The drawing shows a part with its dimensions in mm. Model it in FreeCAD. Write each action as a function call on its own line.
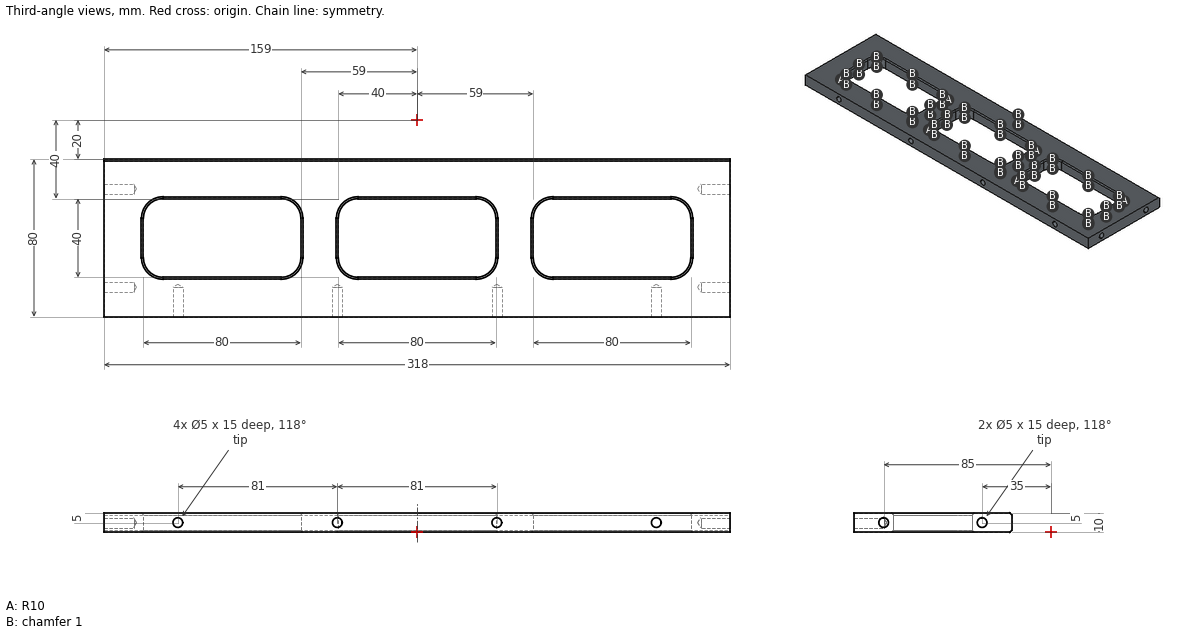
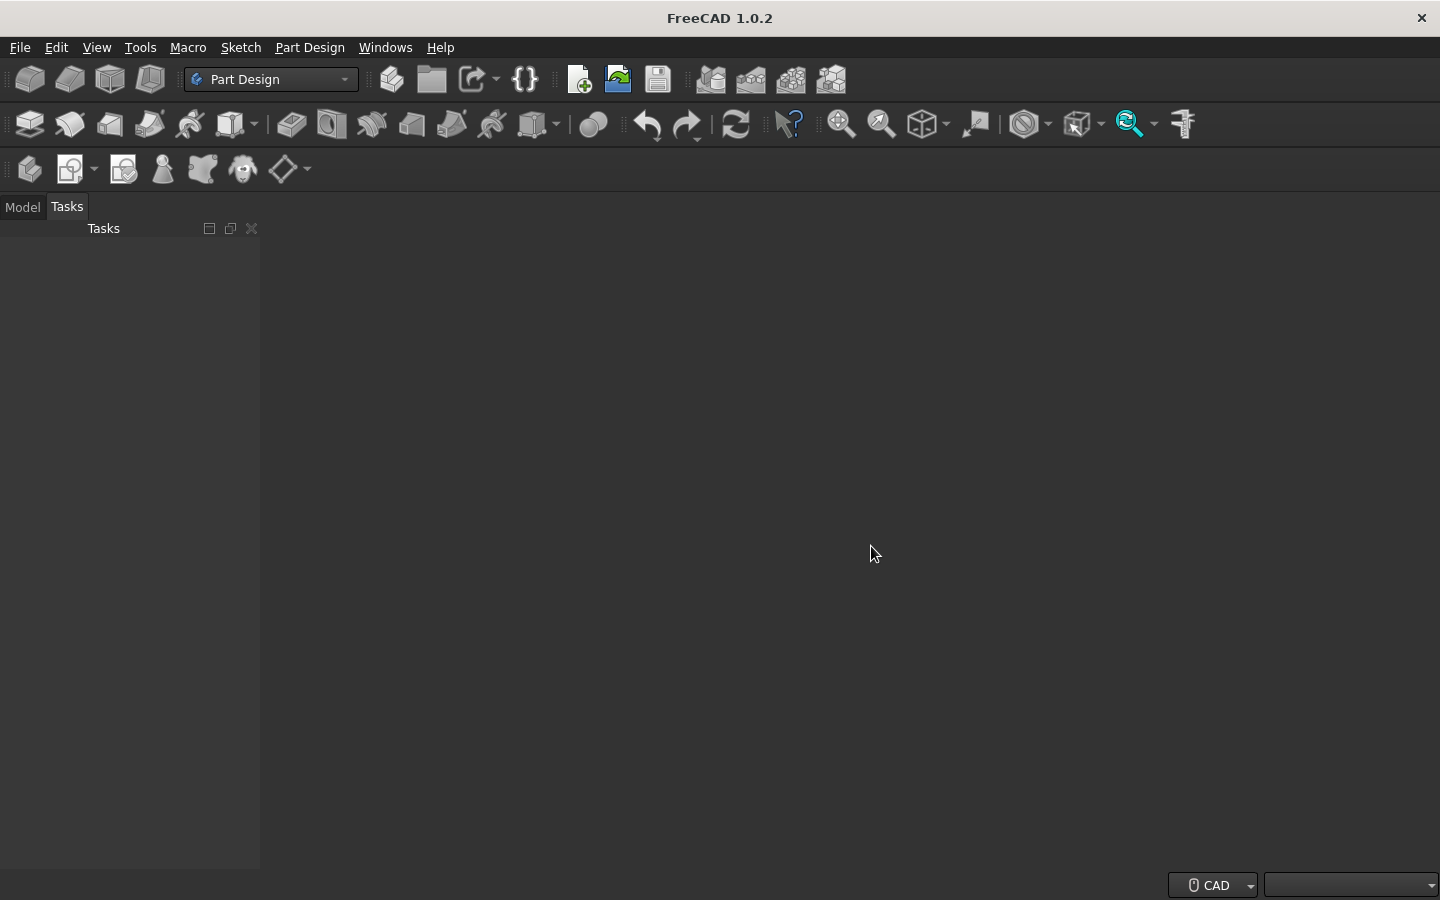
click(578, 80)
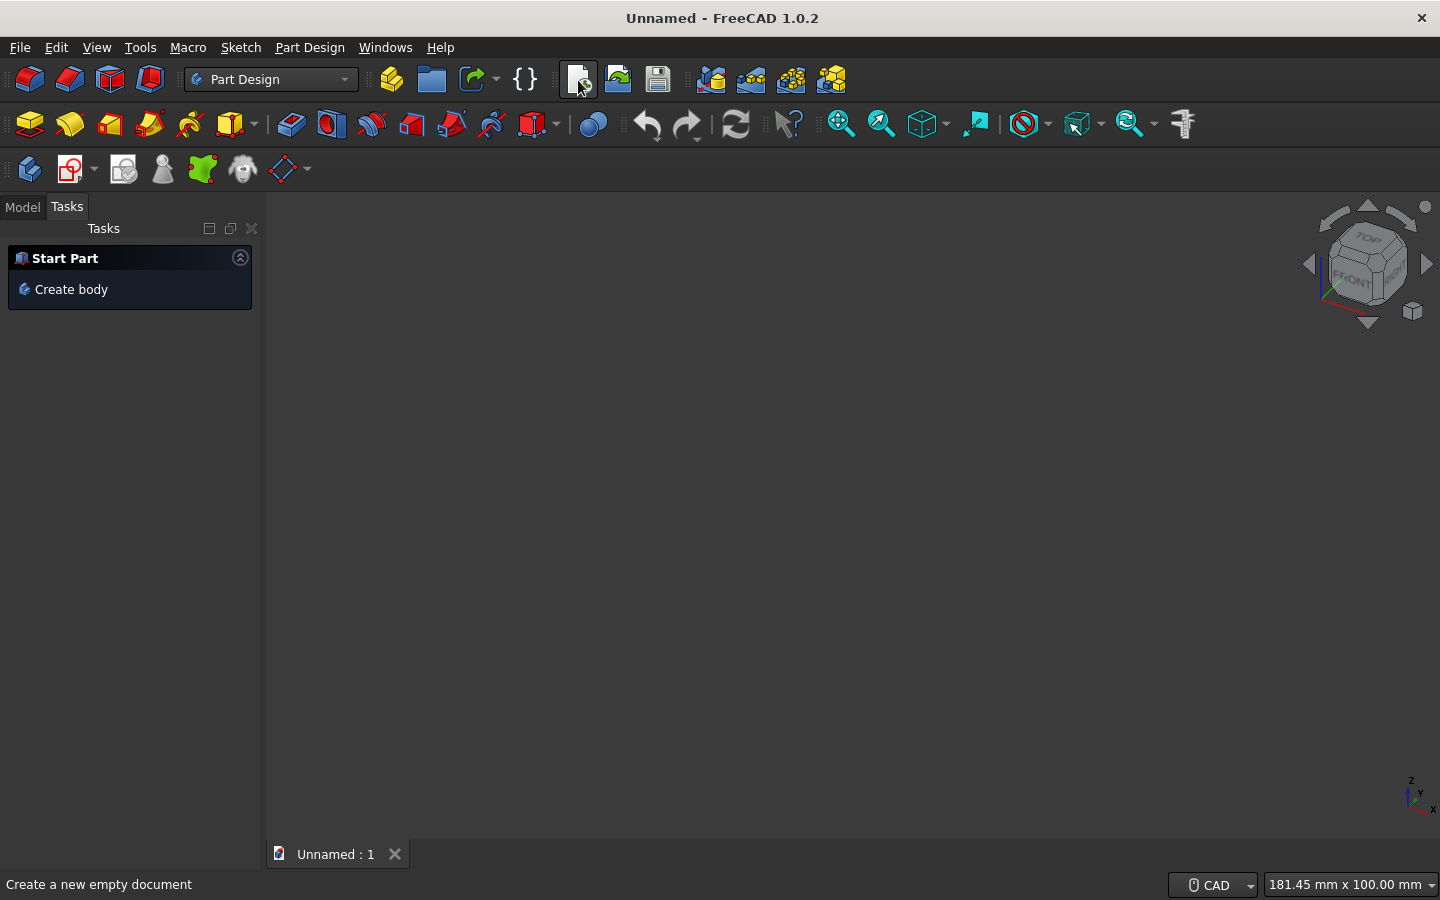
click(30, 170)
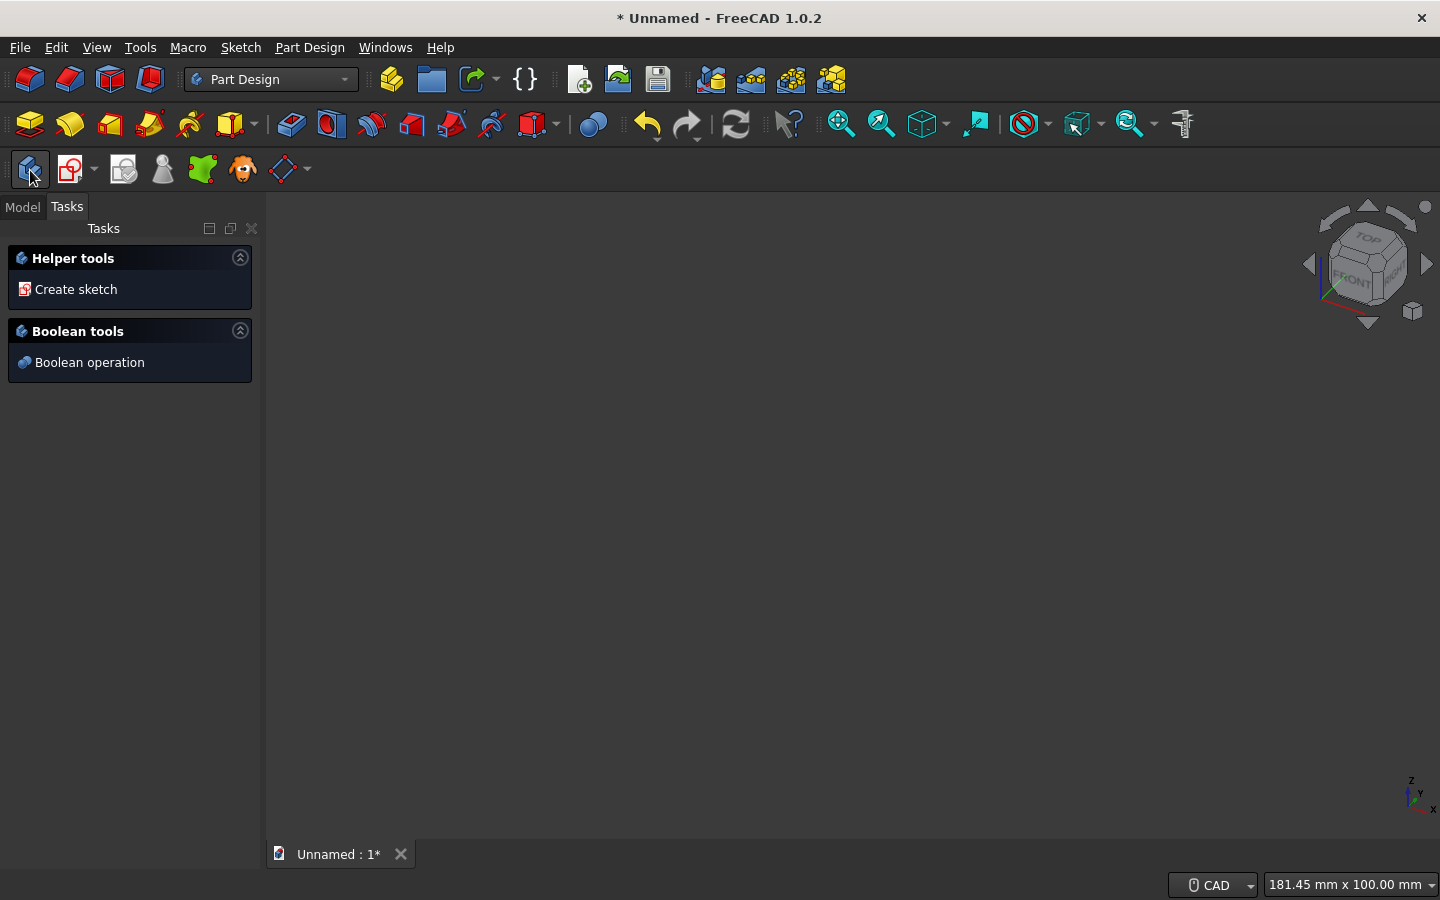
click(23, 206)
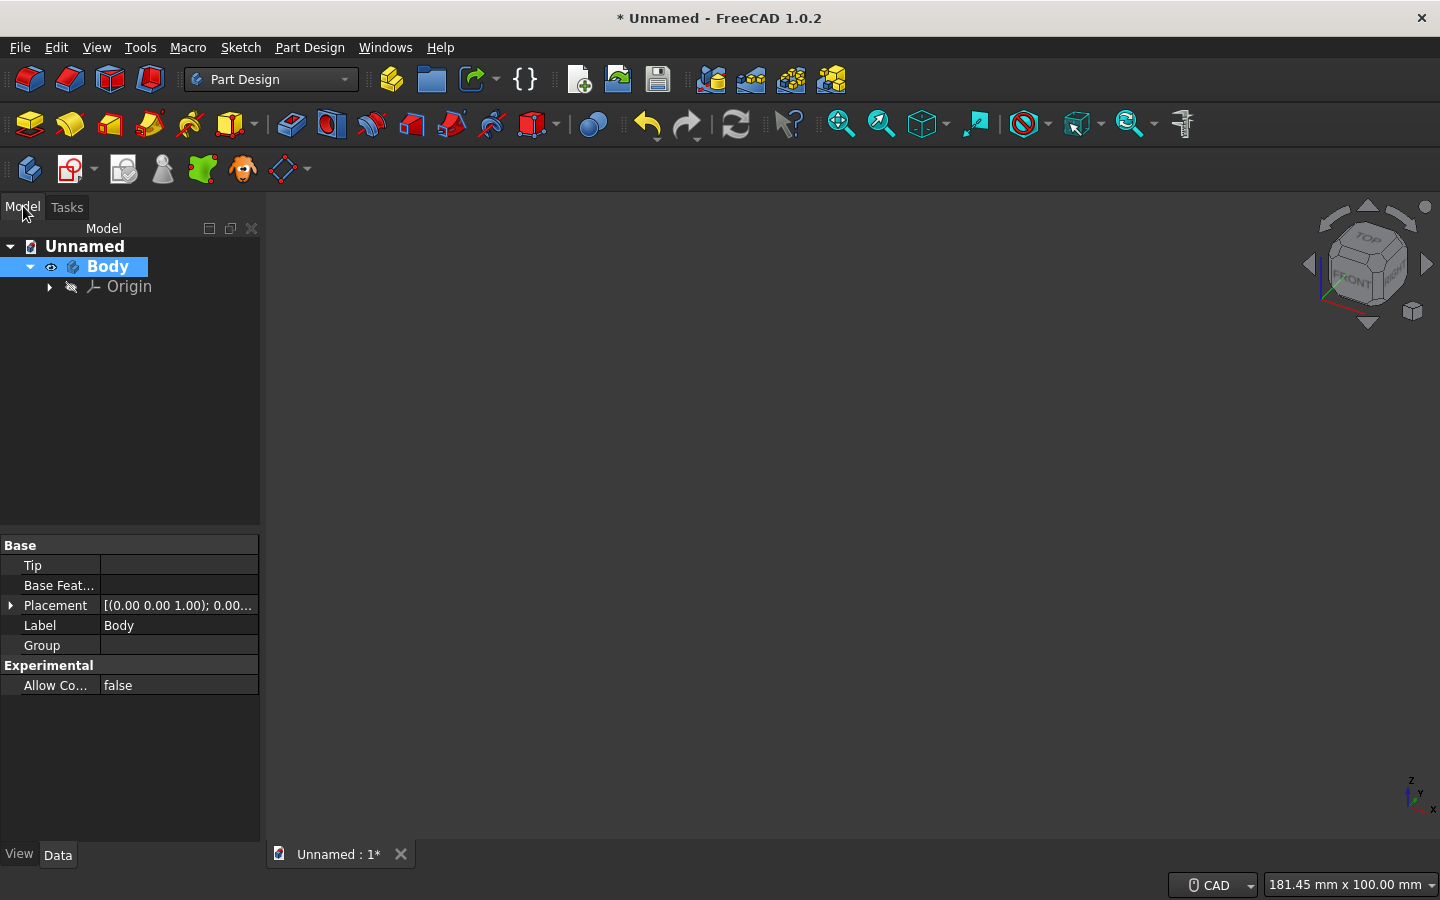
click(50, 287)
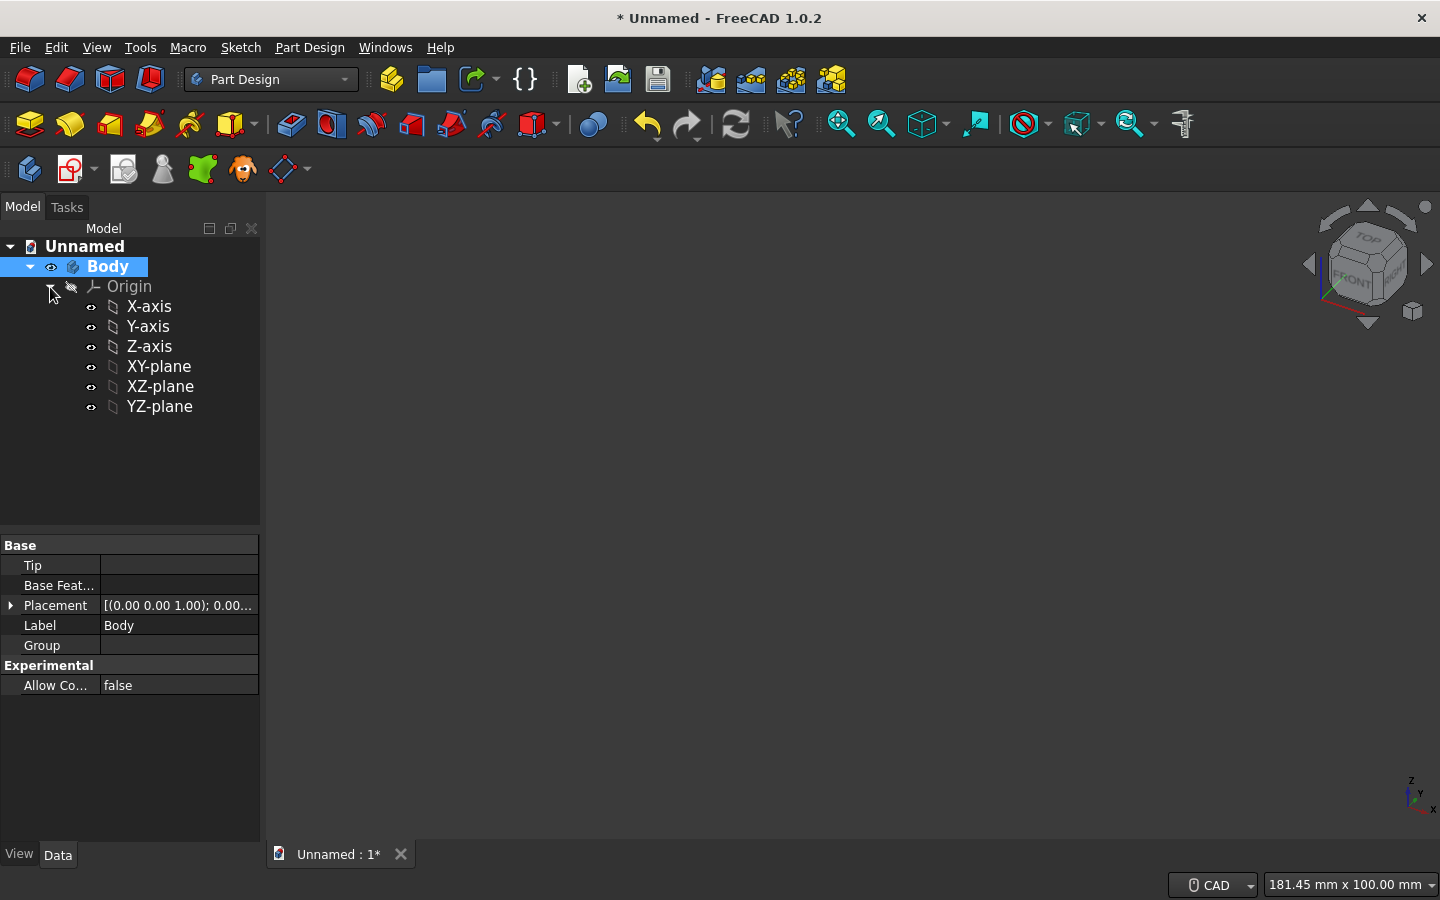
click(136, 367)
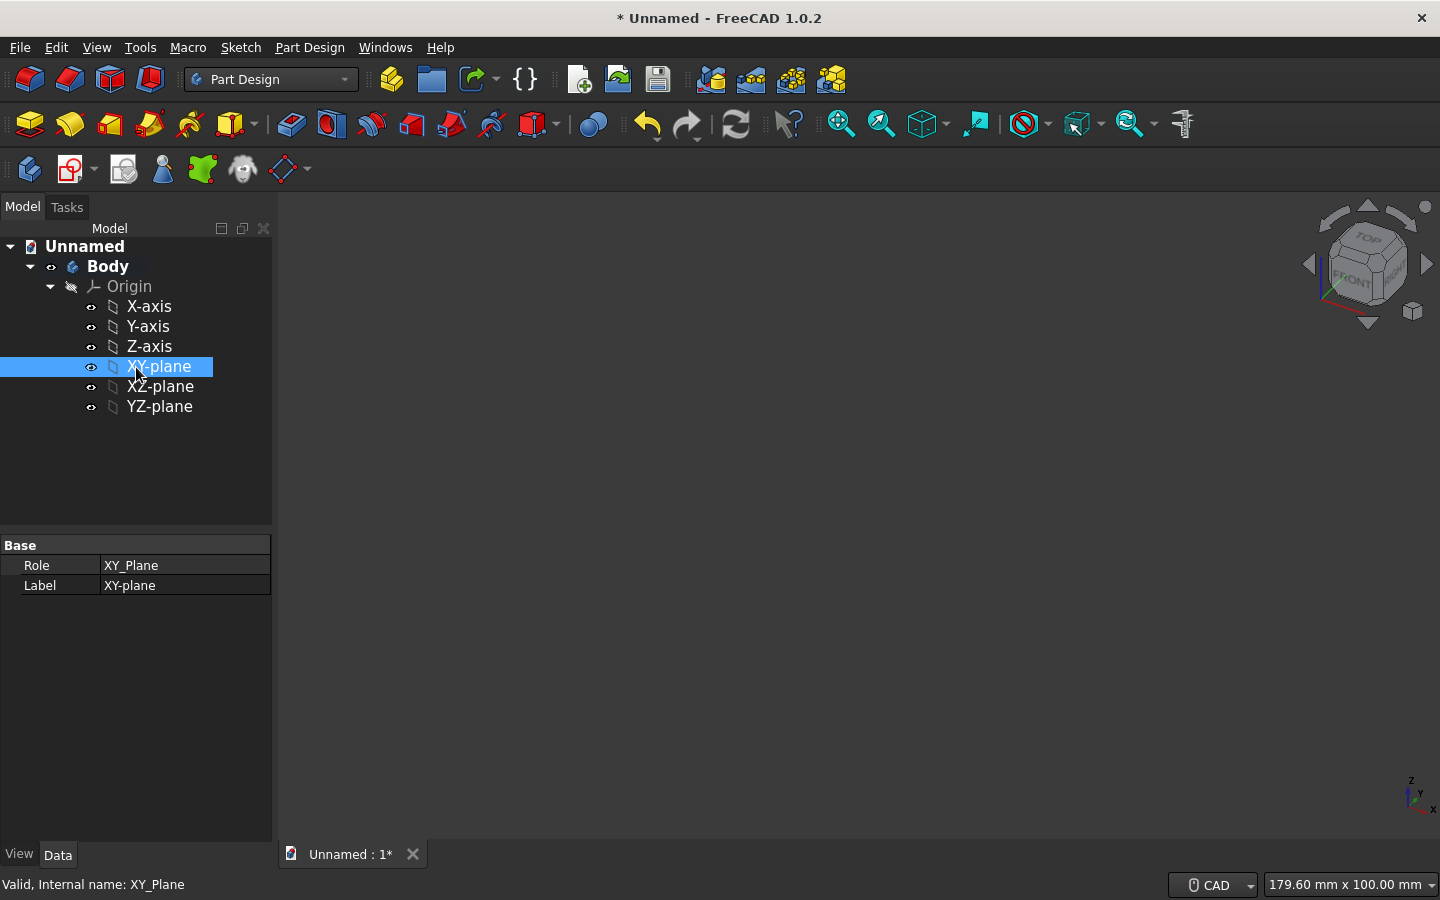
click(284, 170)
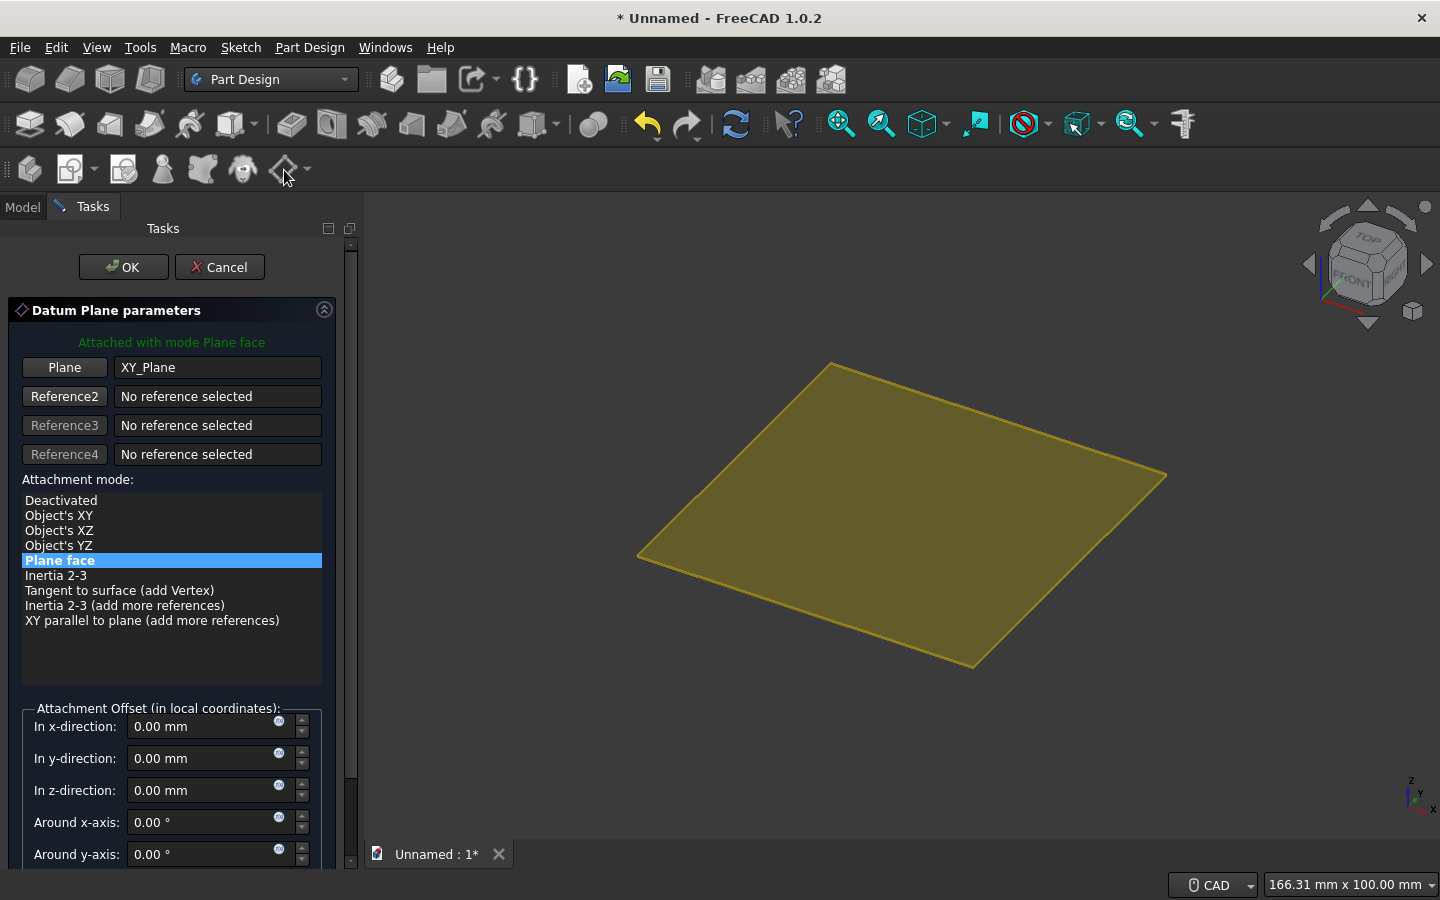
triple_click(210, 790)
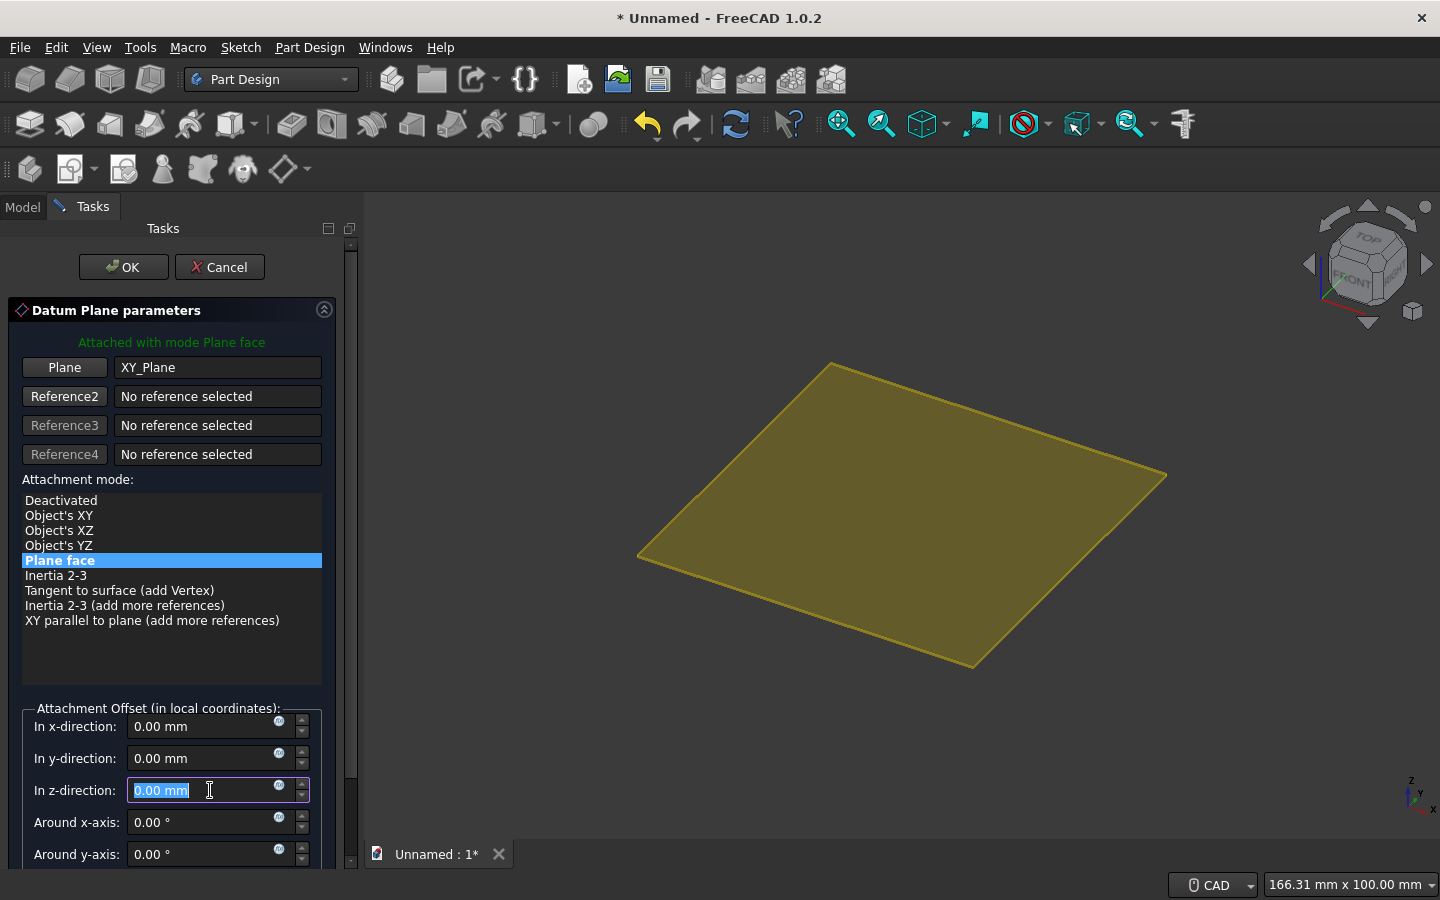
text(10)
key(Tab)